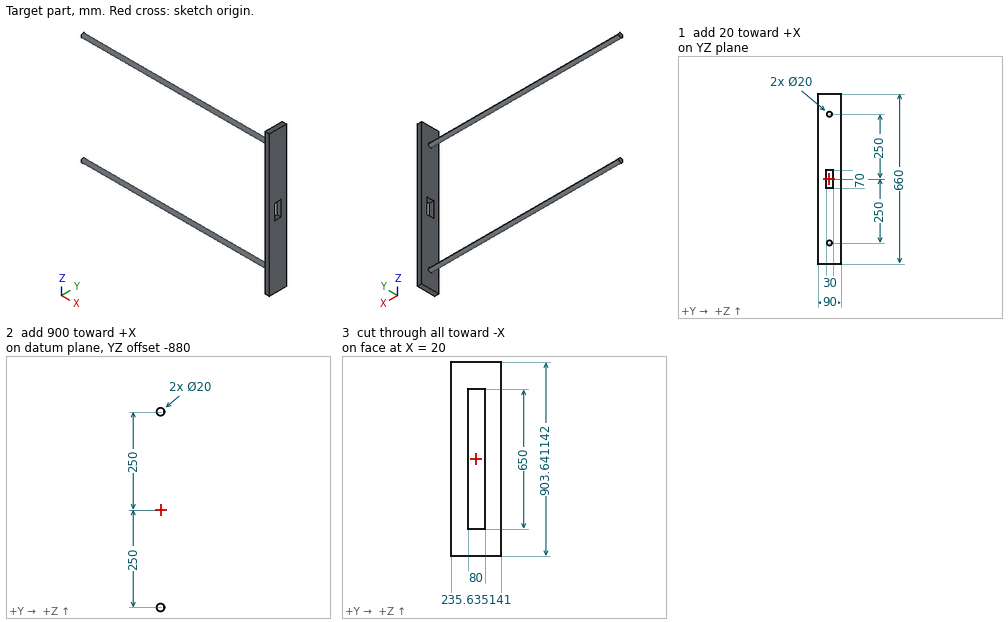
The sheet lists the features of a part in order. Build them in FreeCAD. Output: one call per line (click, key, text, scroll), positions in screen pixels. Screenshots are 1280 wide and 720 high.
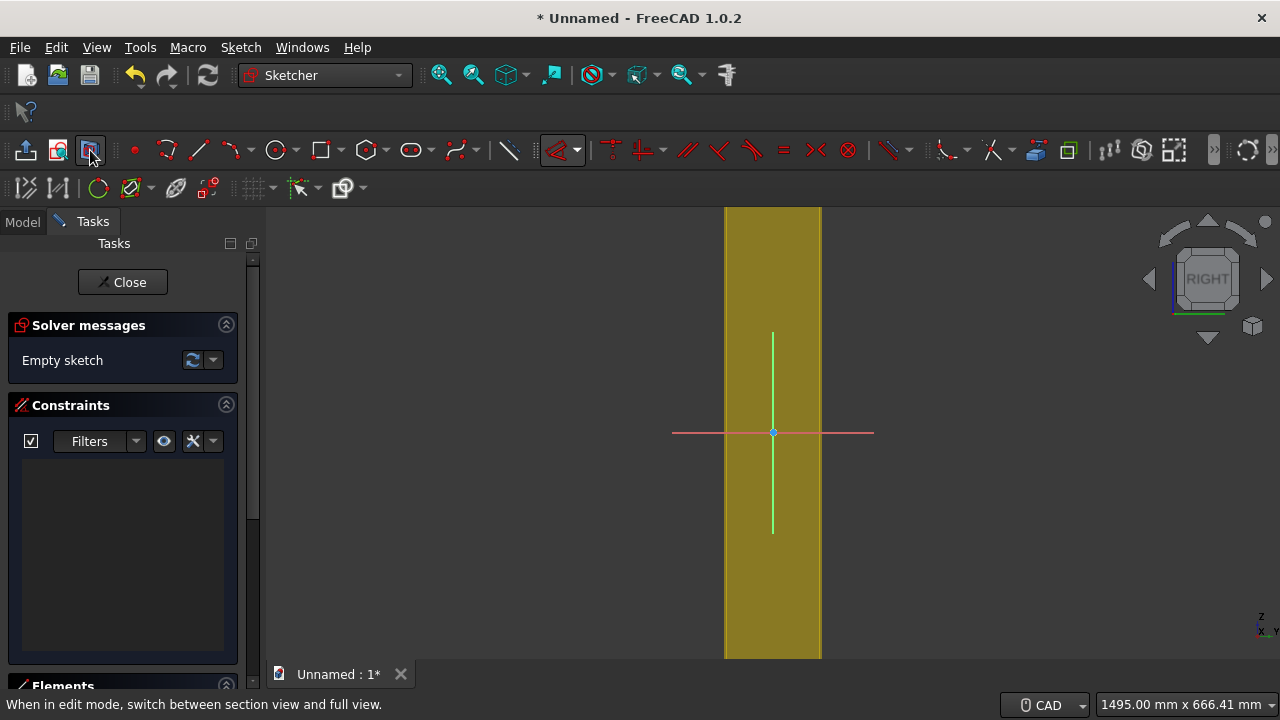
scroll(395, 433, down, 1)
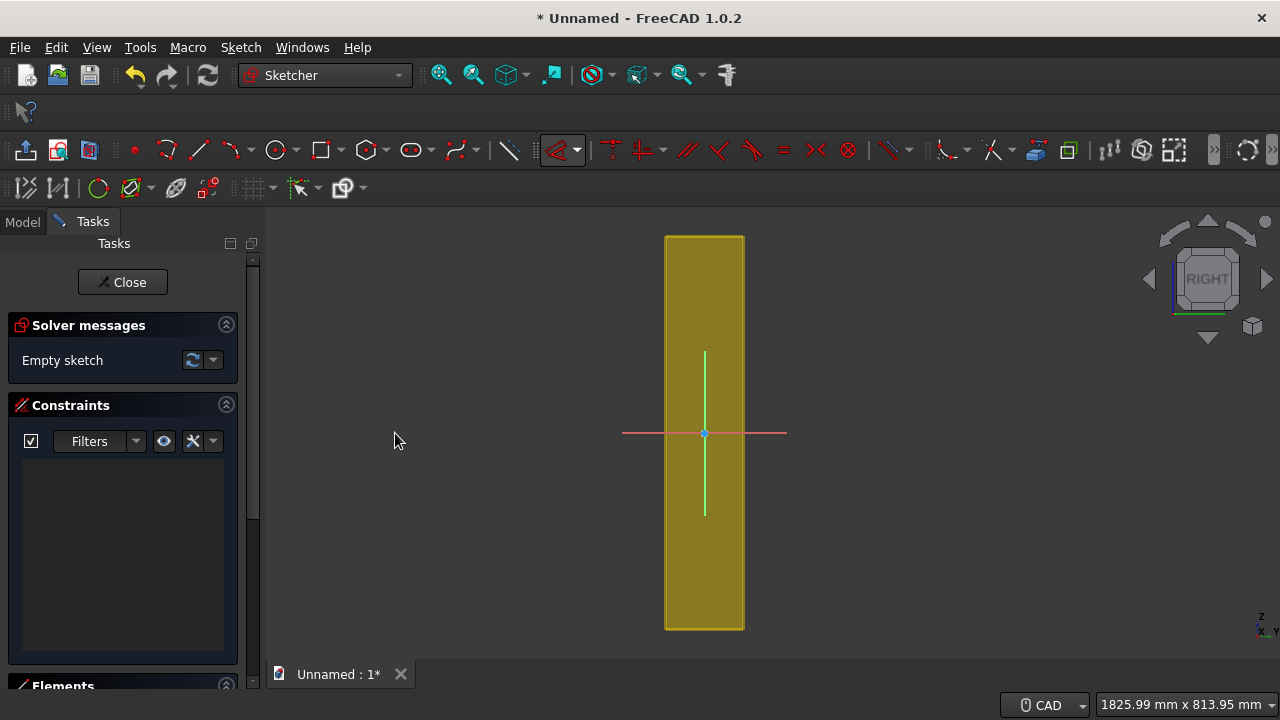
click(276, 150)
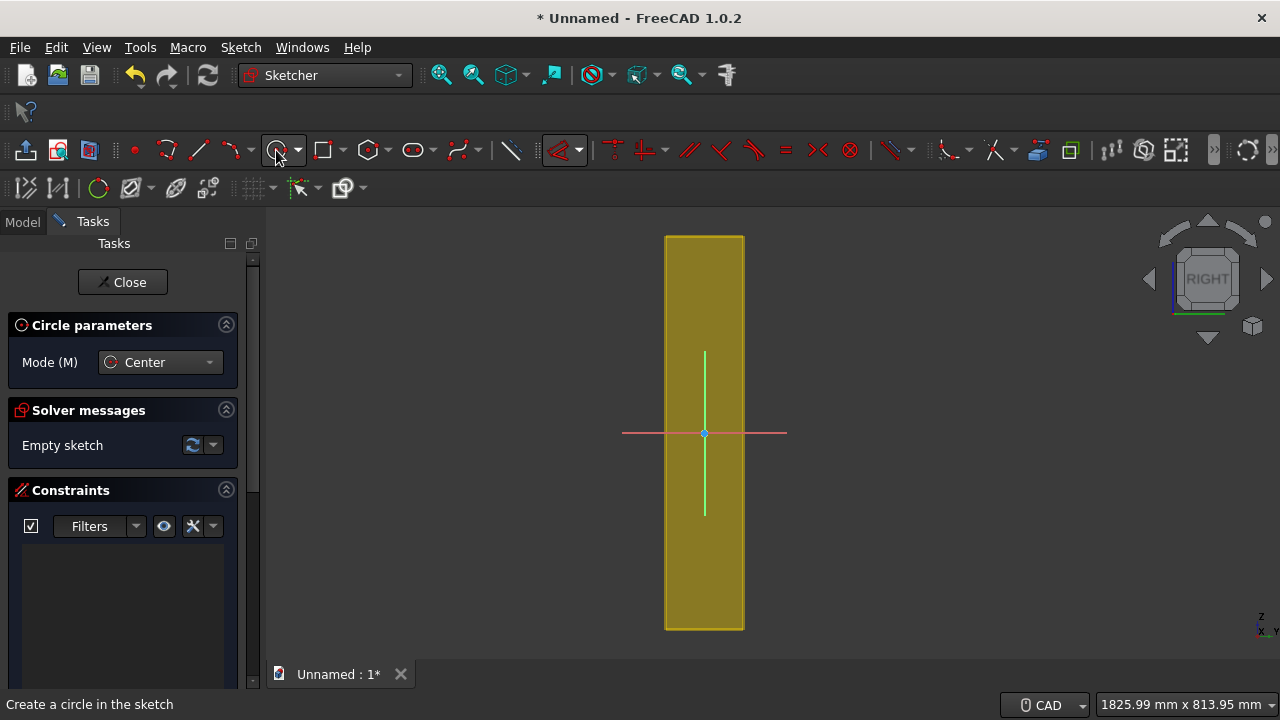
scroll(705, 294, up, 8)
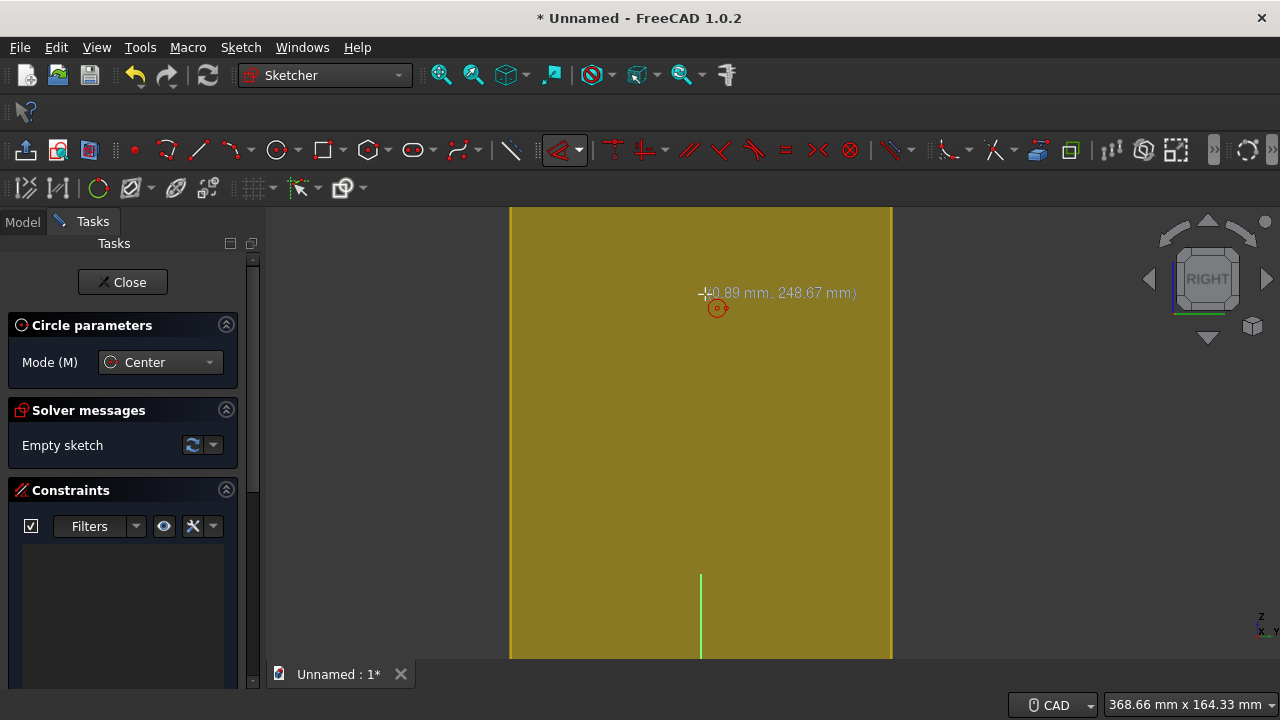
scroll(705, 294, down, 8)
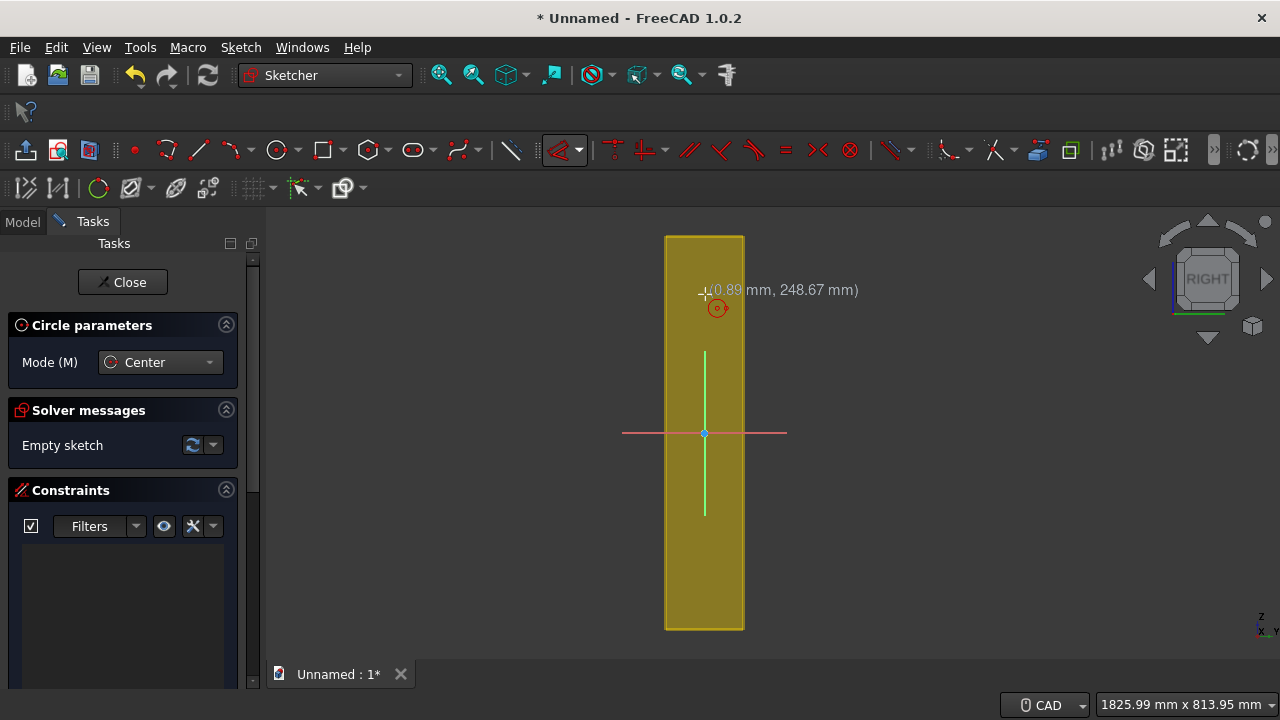
click(705, 294)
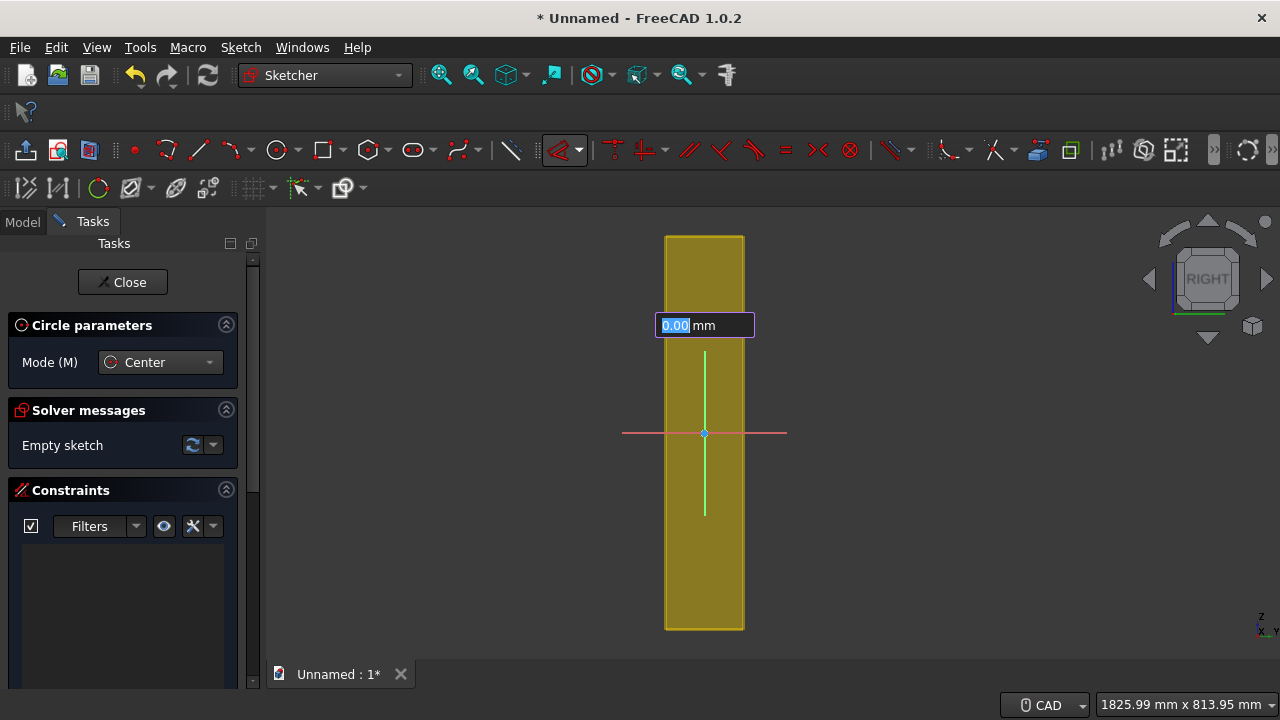
scroll(710, 292, up, 6)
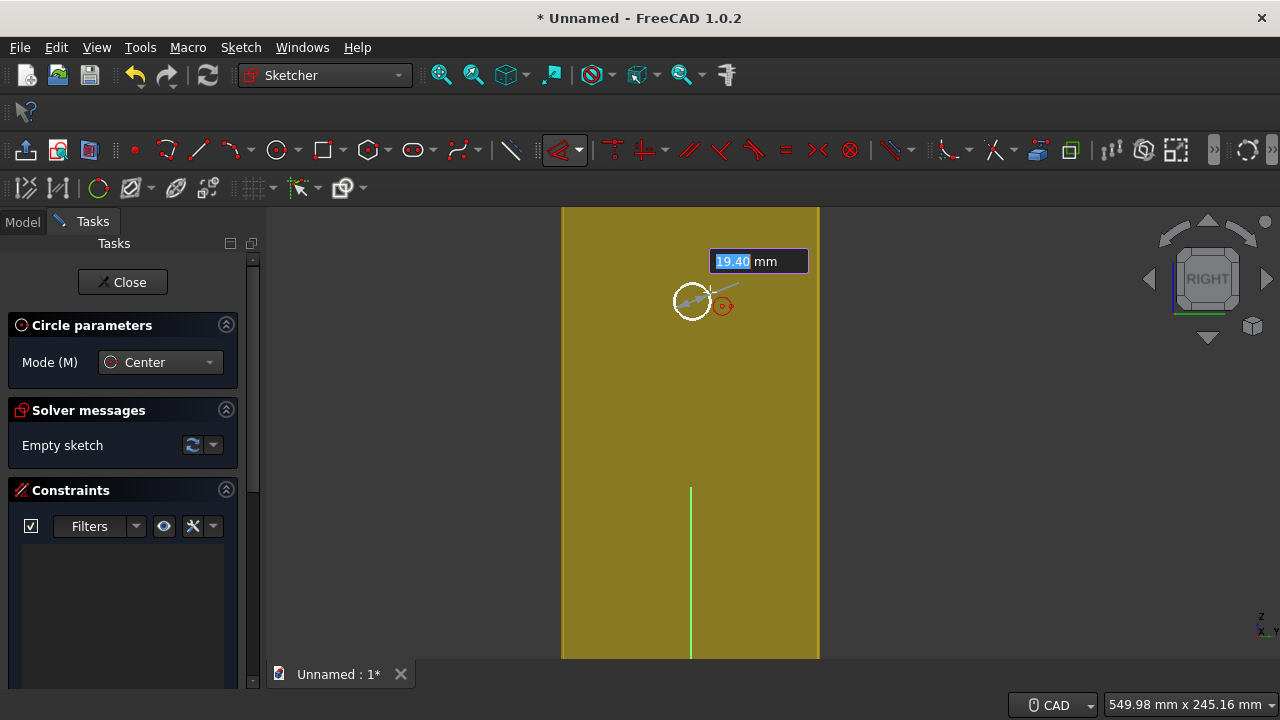
click(708, 293)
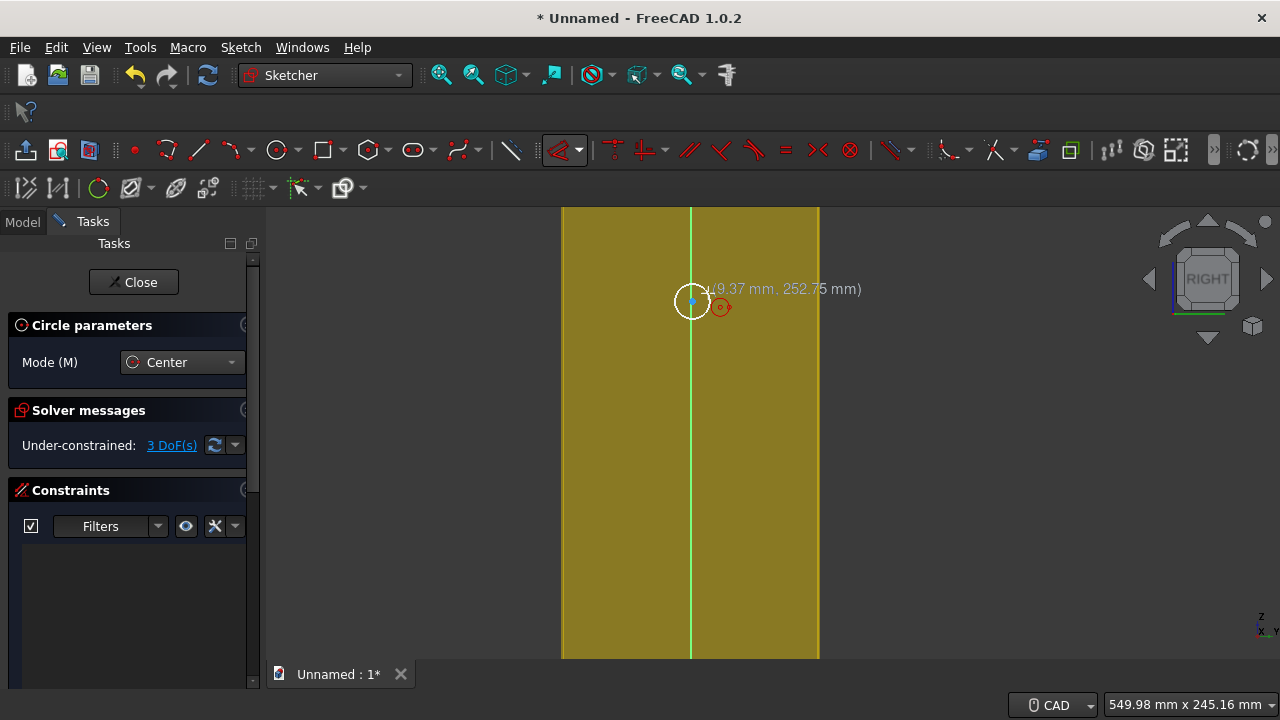
scroll(710, 292, down, 6)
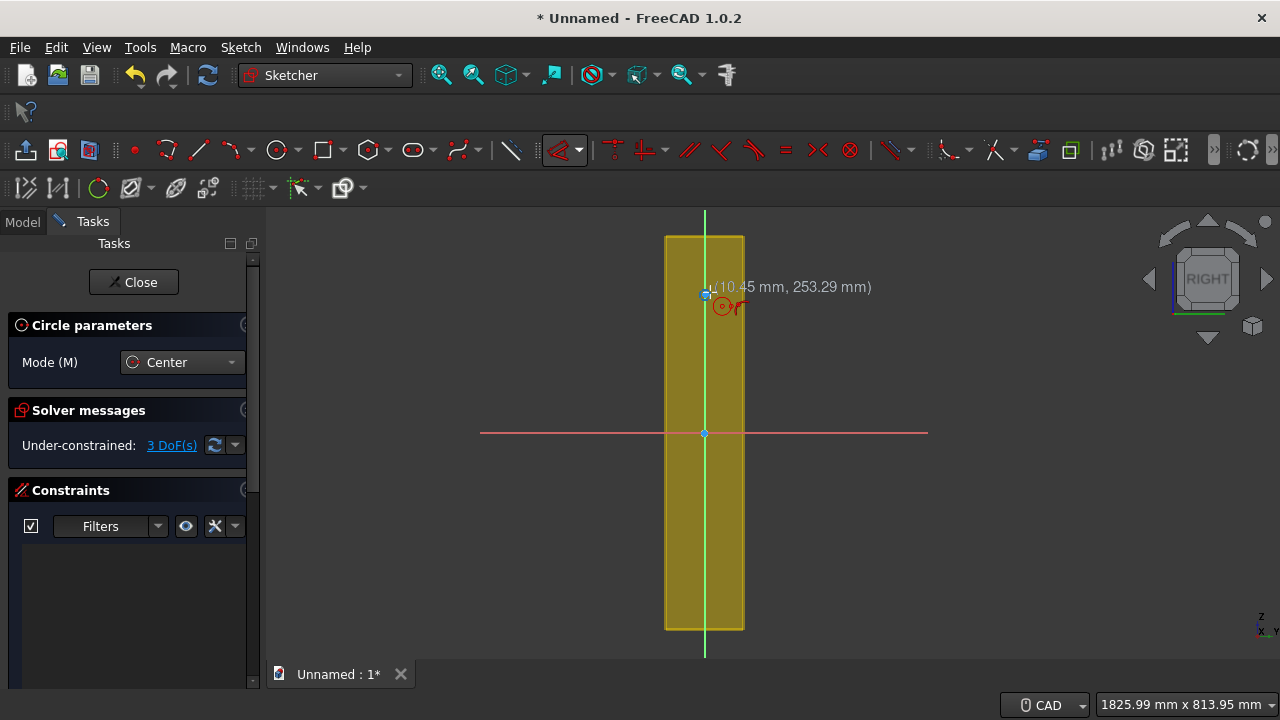
scroll(705, 572, up, 8)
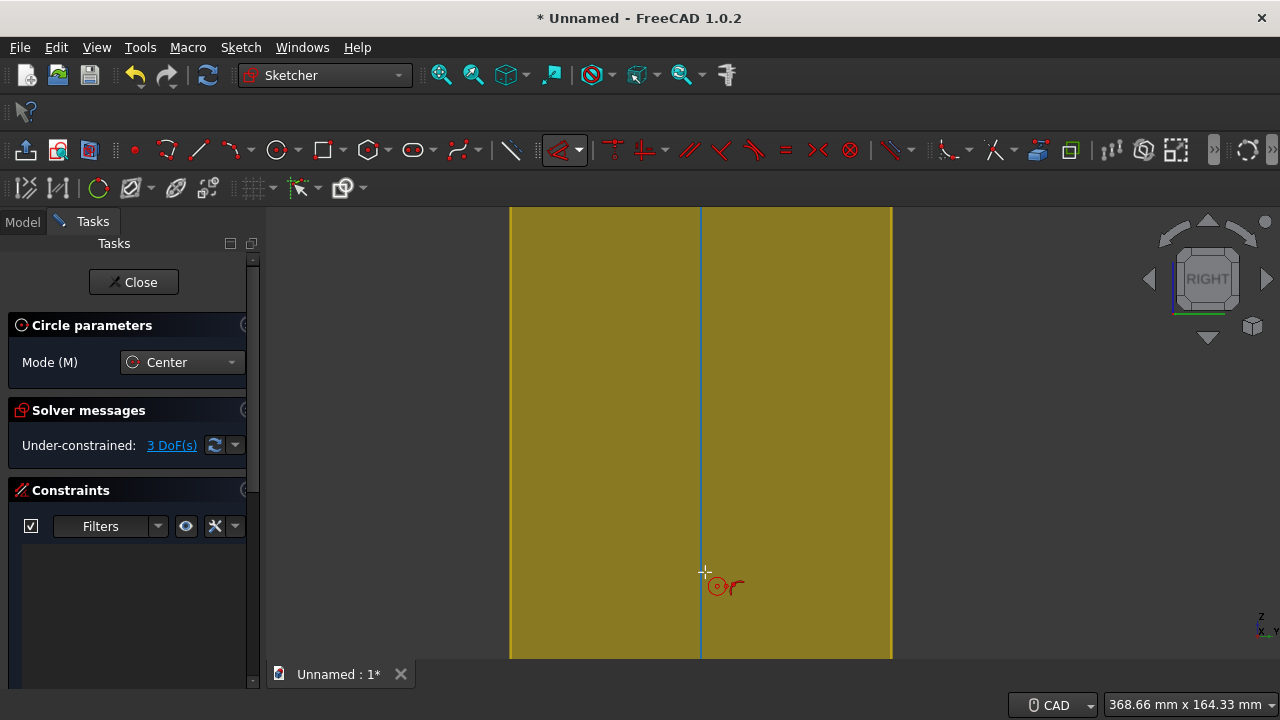
scroll(705, 573, down, 8)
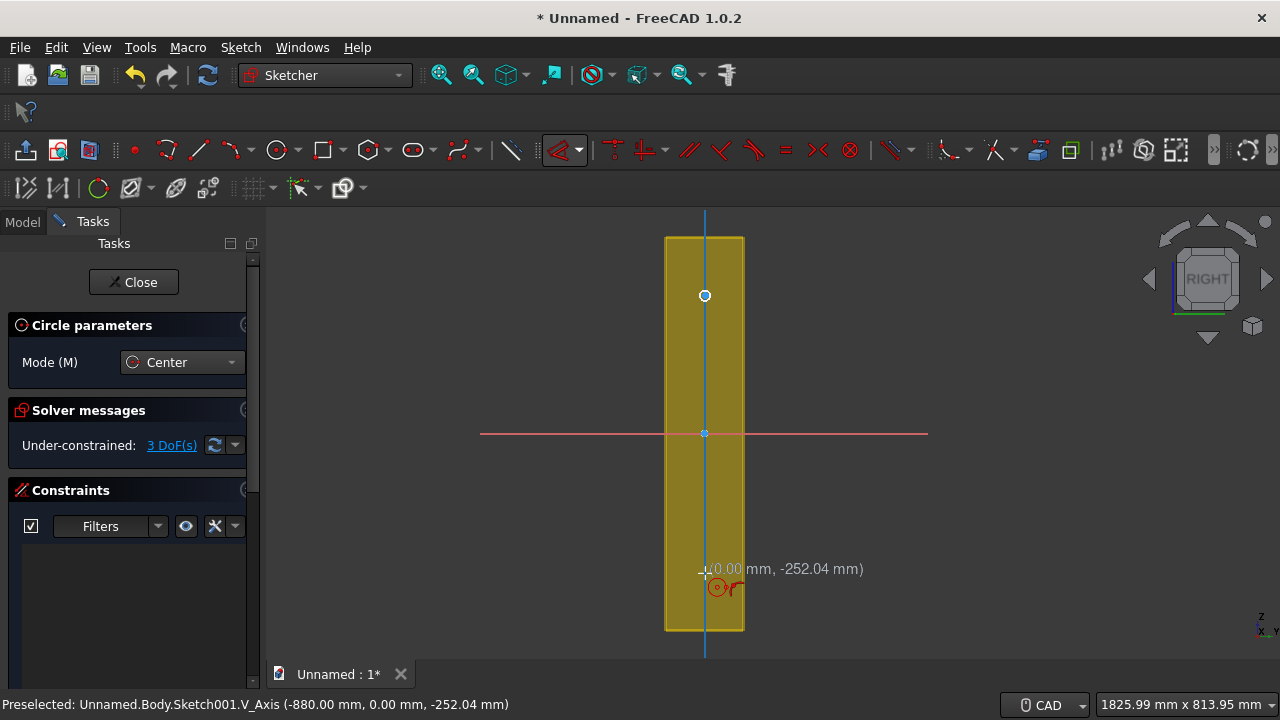
click(705, 573)